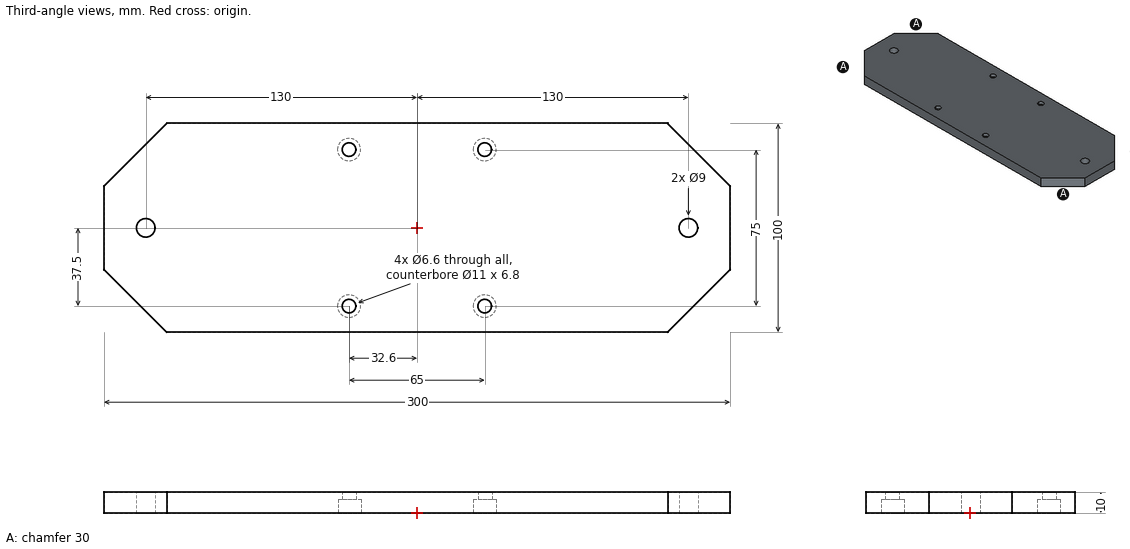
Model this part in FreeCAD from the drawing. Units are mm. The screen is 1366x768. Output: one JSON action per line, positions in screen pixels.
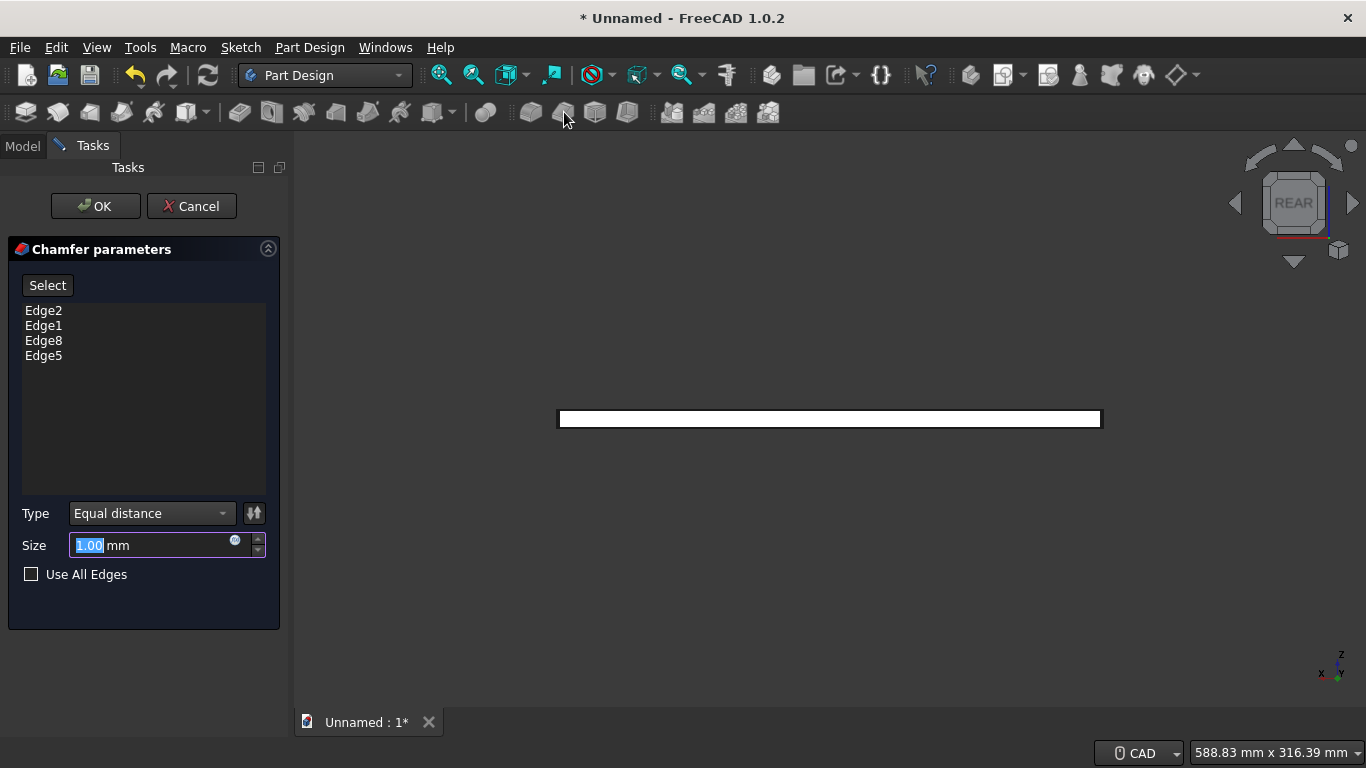
{"action": "type", "text": "30"}
{"action": "key", "text": "Tab"}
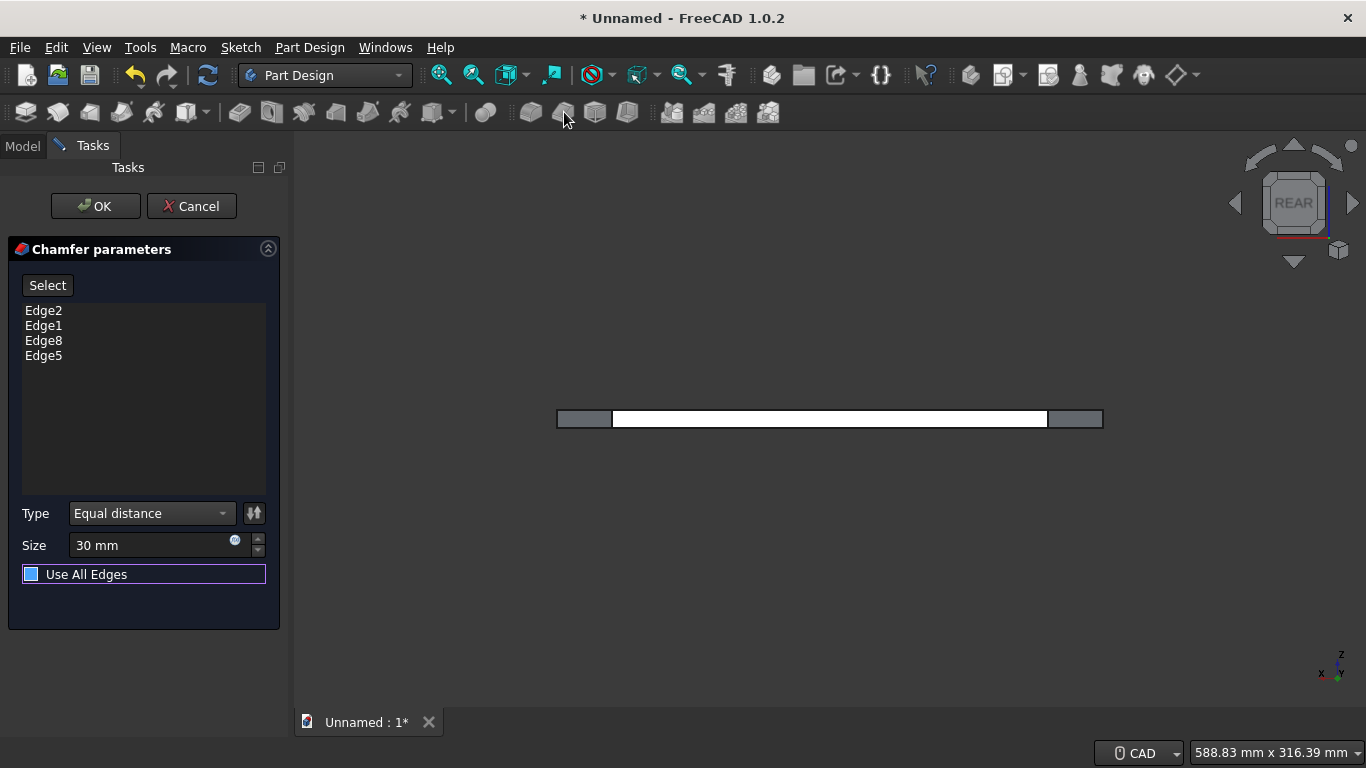
{"action": "left_click", "coordinate": [96, 206]}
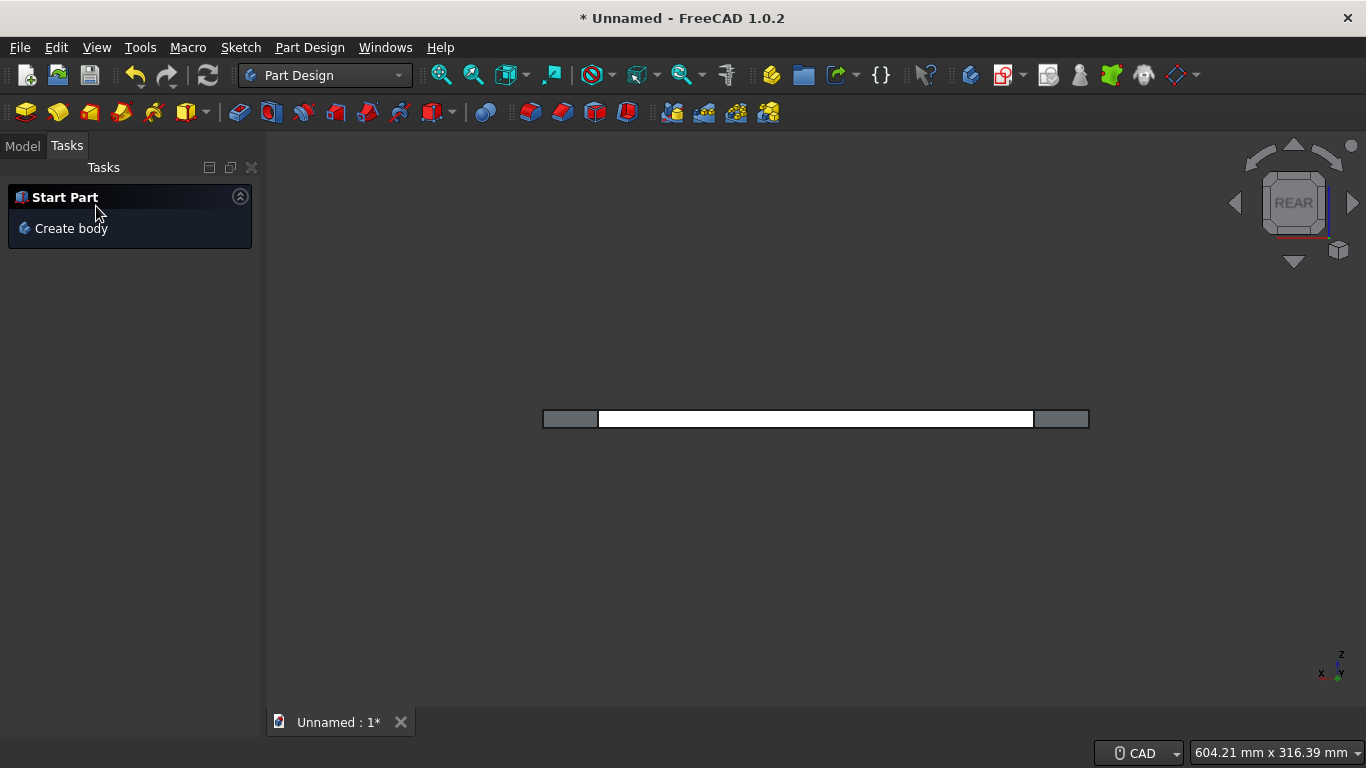
{"action": "key", "text": "0"}